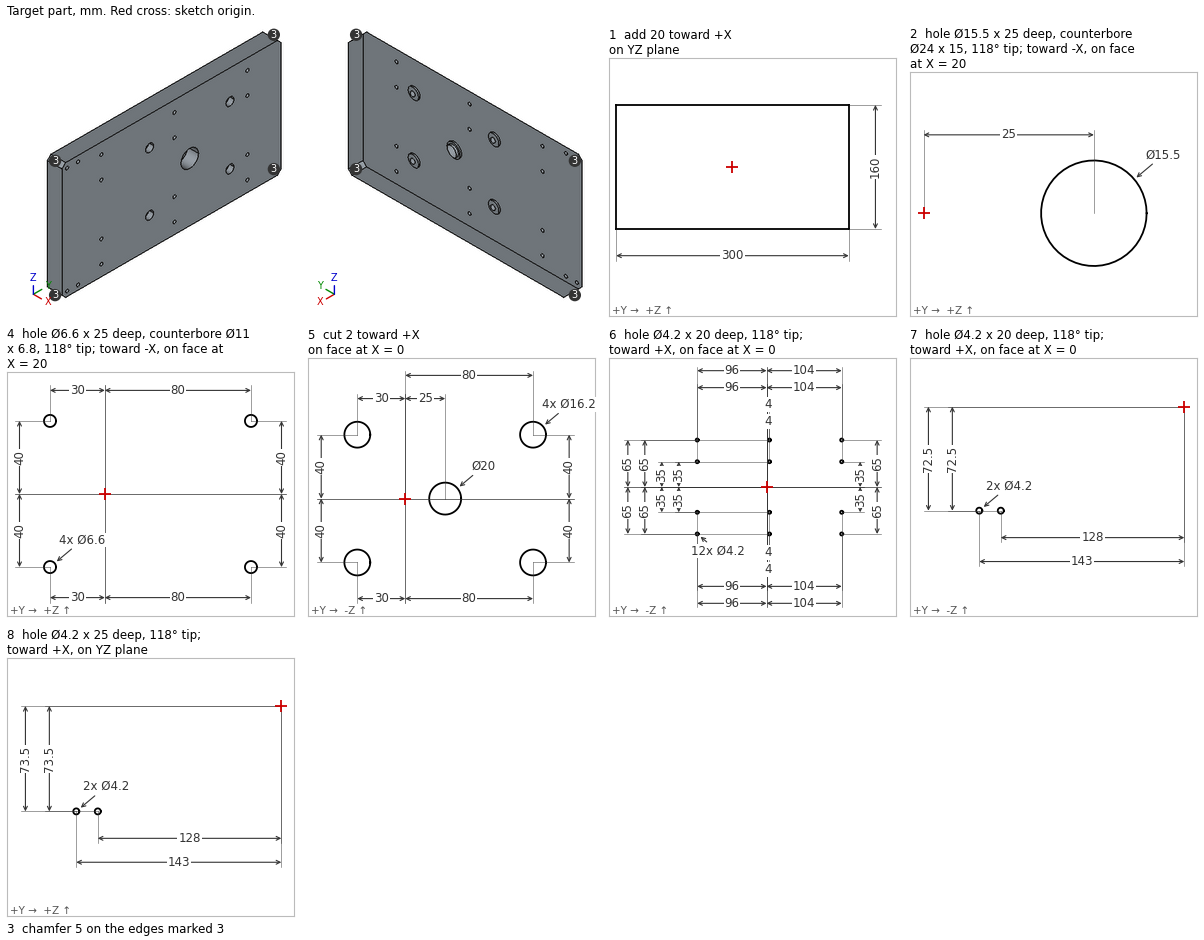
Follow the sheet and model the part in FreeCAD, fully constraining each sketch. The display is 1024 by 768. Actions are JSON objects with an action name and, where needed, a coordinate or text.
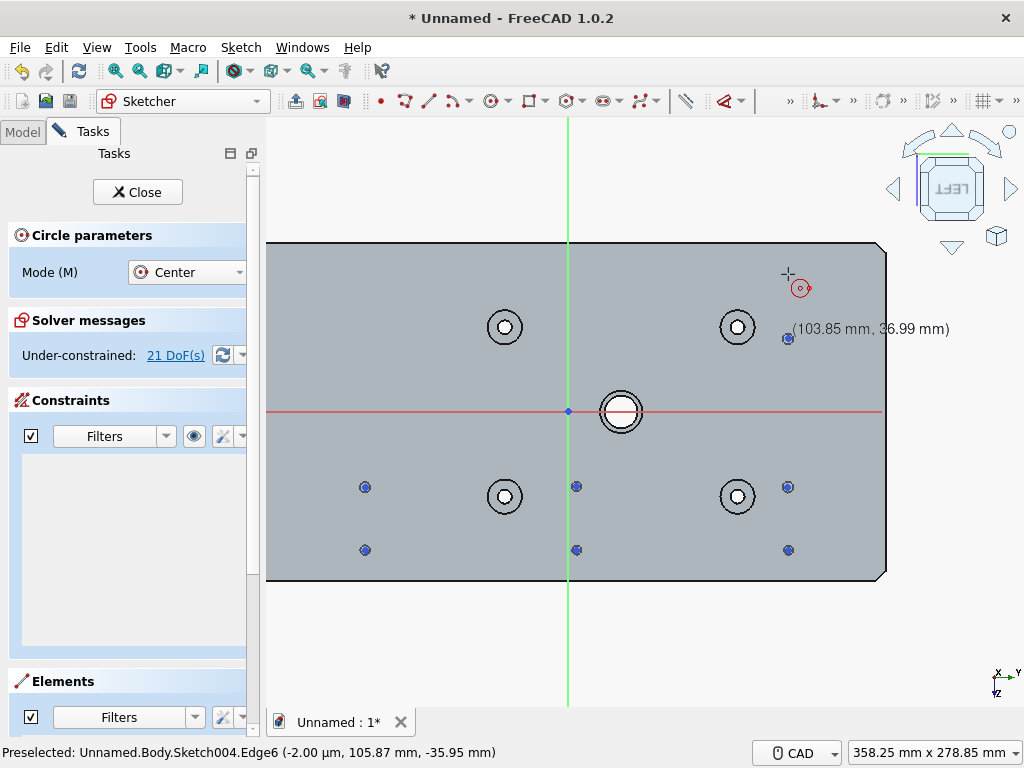
{"action": "left_click", "coordinate": [788, 274]}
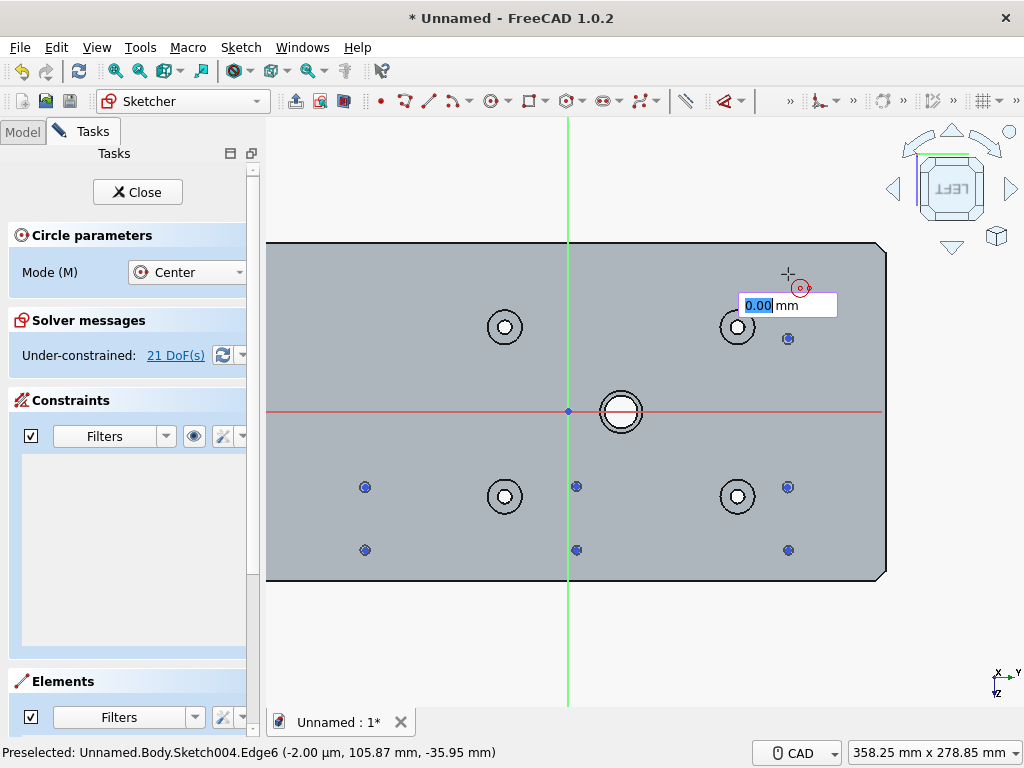
{"action": "scroll", "coordinate": [791, 271], "scroll_direction": "up", "scroll_amount": 7}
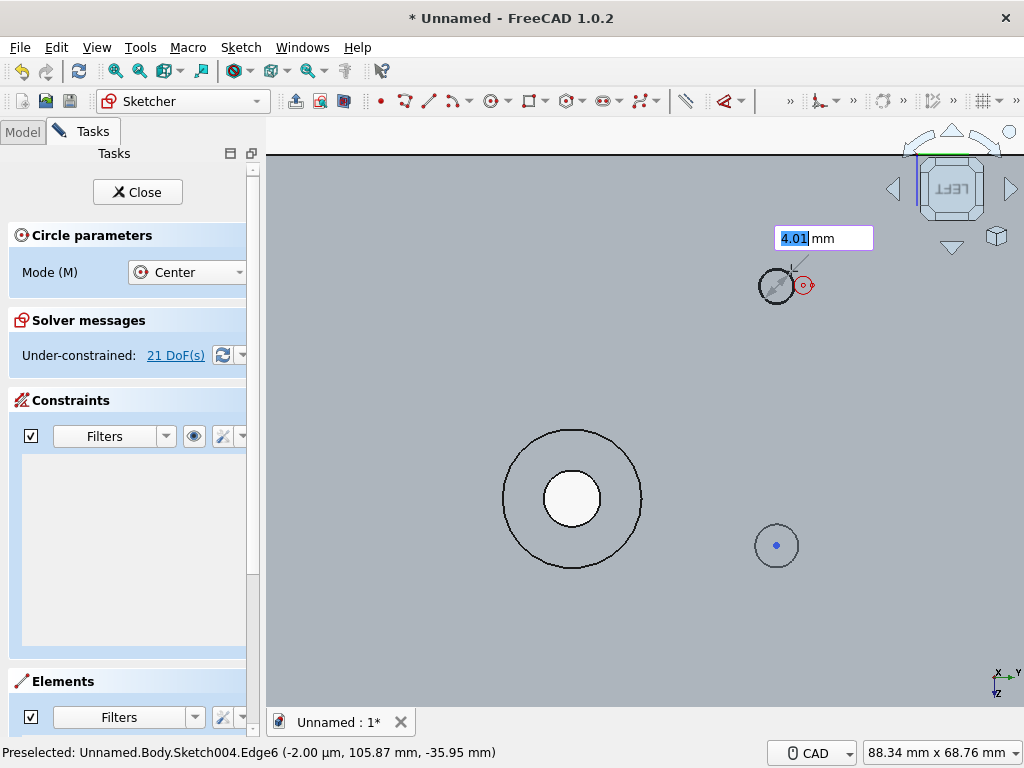
{"action": "left_click", "coordinate": [791, 271]}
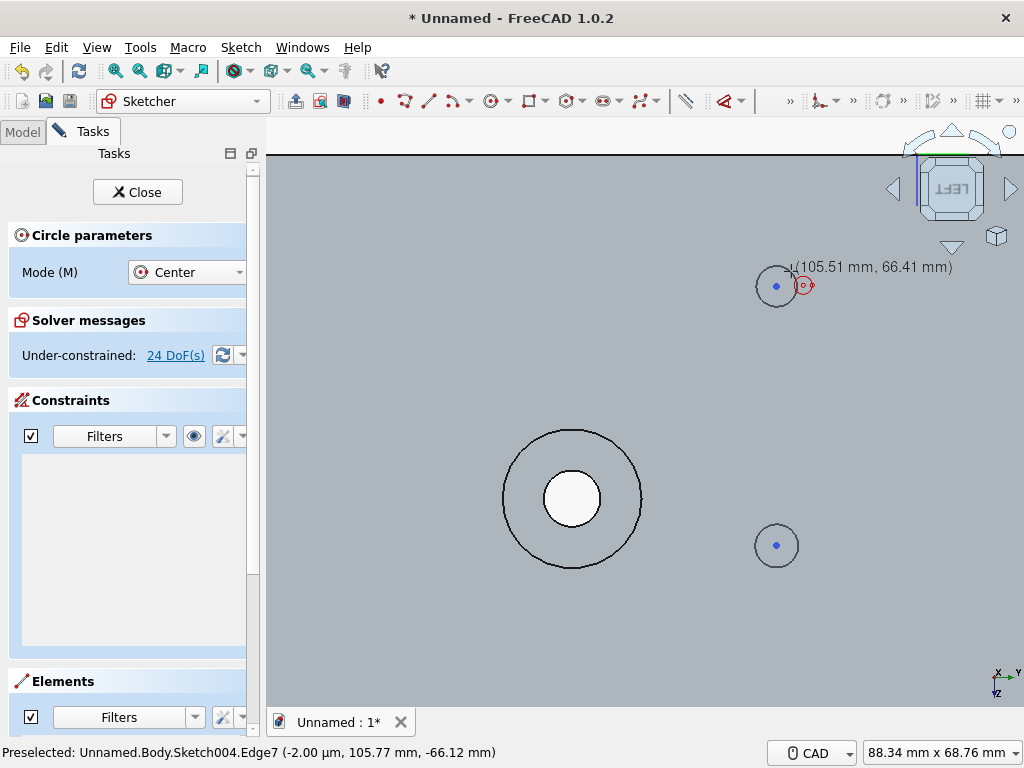
{"action": "scroll", "coordinate": [791, 271], "scroll_direction": "down", "scroll_amount": 7}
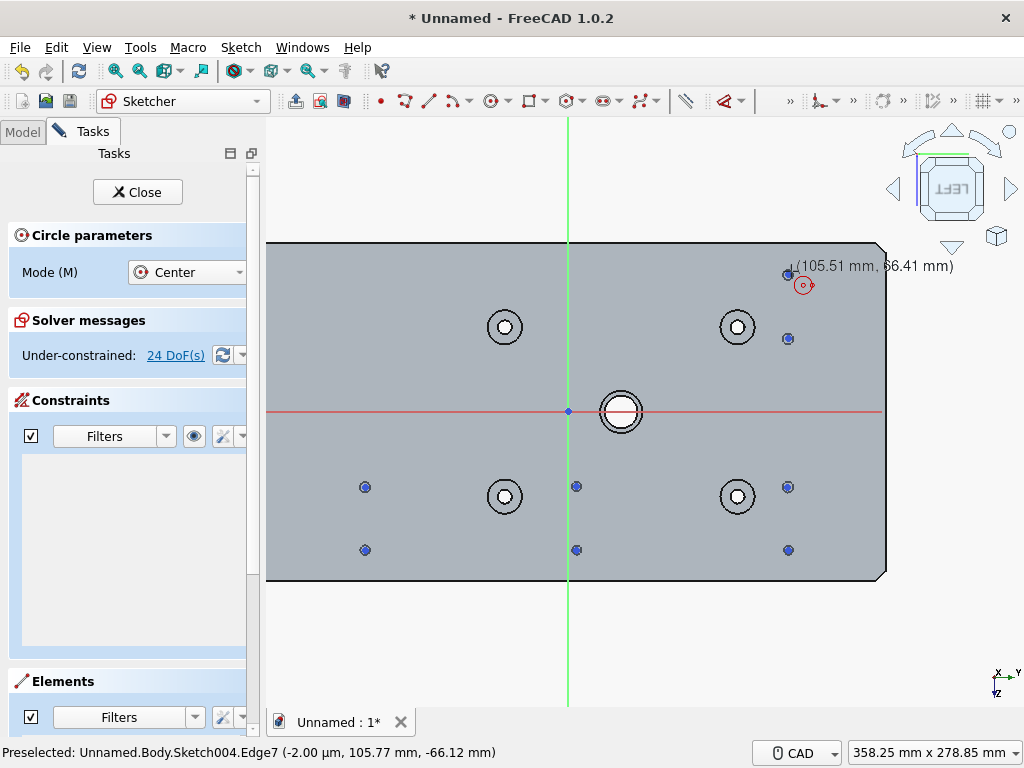
{"action": "scroll", "coordinate": [577, 338], "scroll_direction": "up", "scroll_amount": 9}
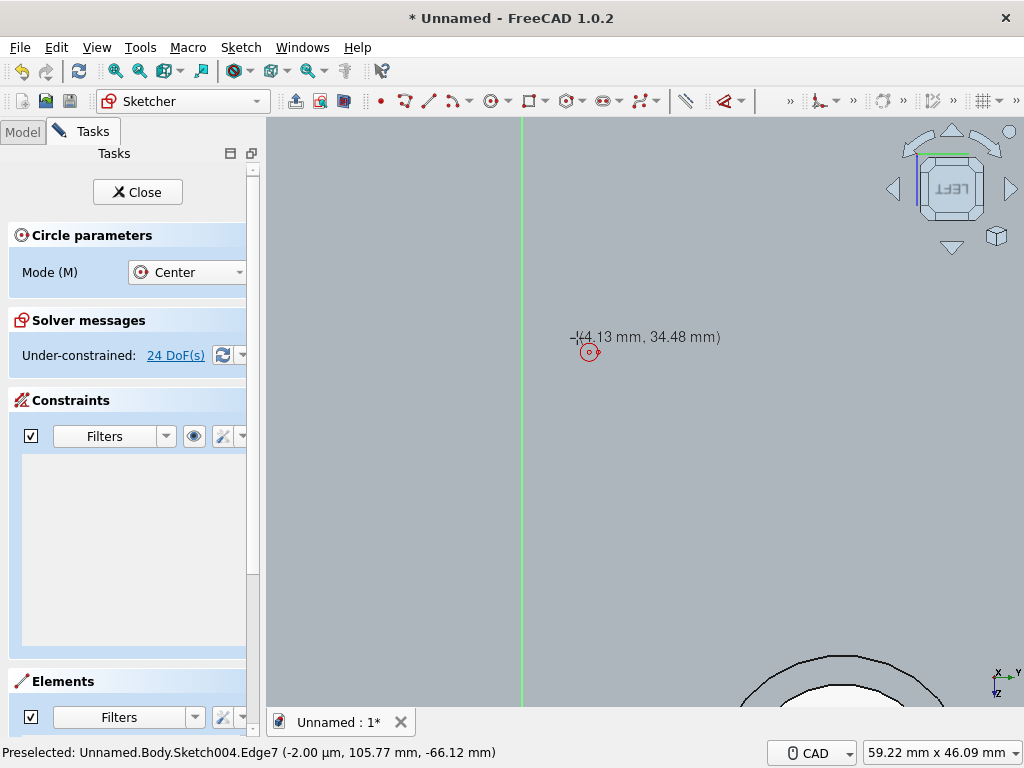
{"action": "scroll", "coordinate": [577, 338], "scroll_direction": "down", "scroll_amount": 9}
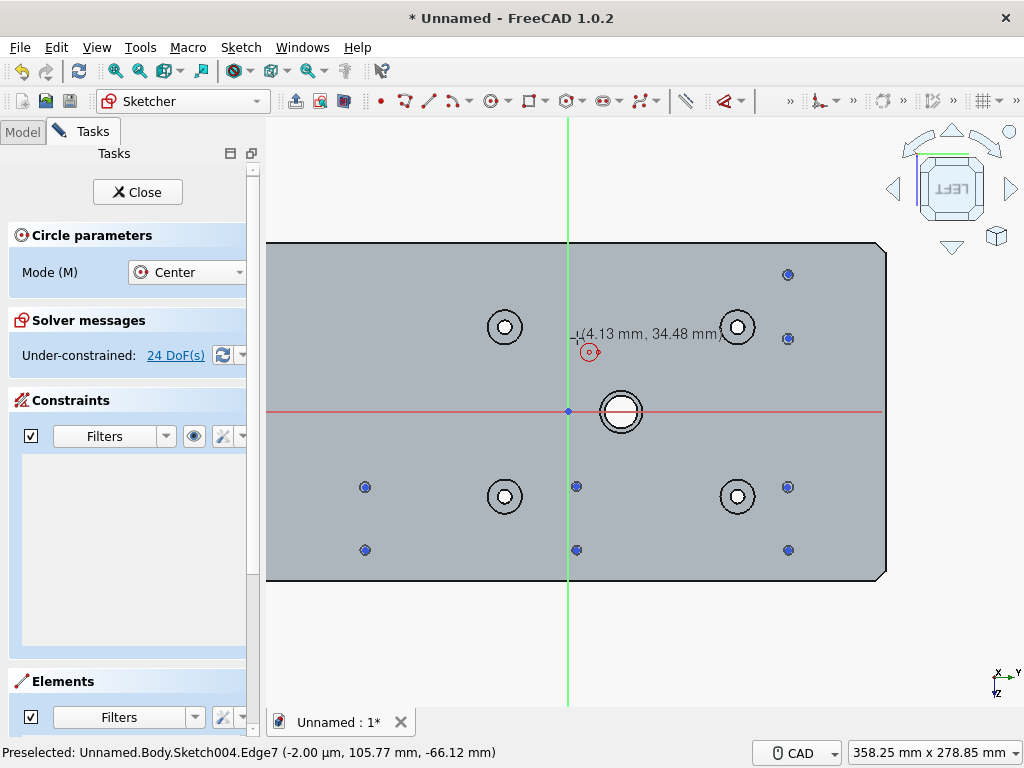
{"action": "scroll", "coordinate": [577, 338], "scroll_direction": "up", "scroll_amount": 4}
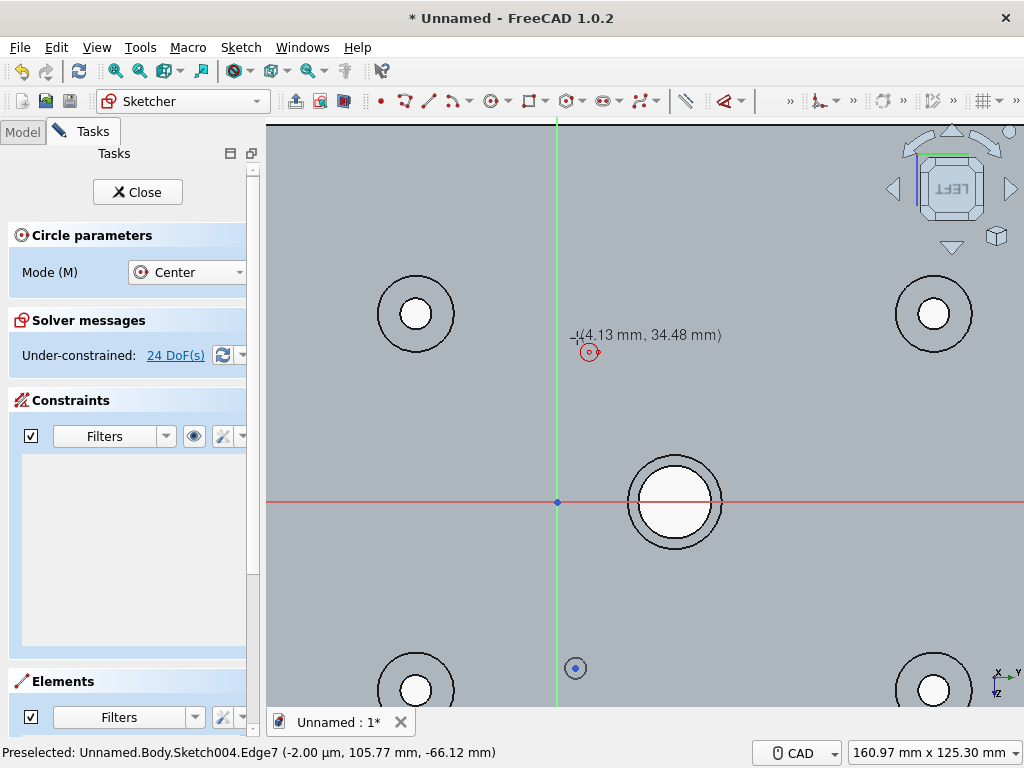
{"action": "left_click", "coordinate": [576, 337]}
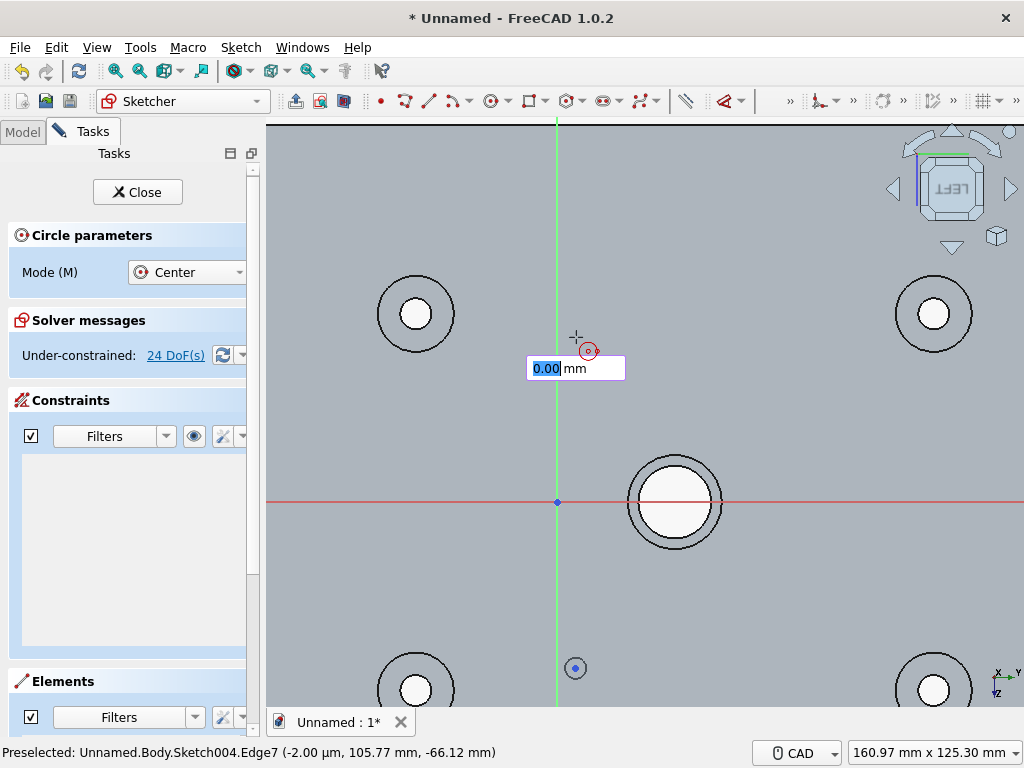
{"action": "scroll", "coordinate": [583, 330], "scroll_direction": "up", "scroll_amount": 3}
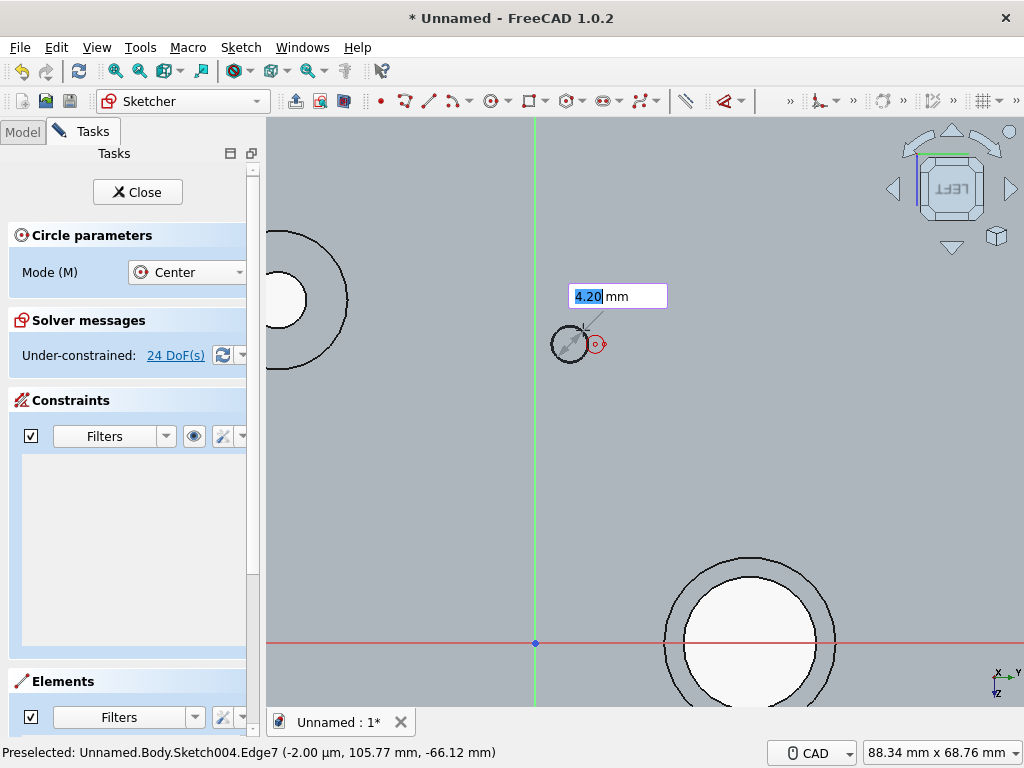
{"action": "left_click", "coordinate": [582, 330]}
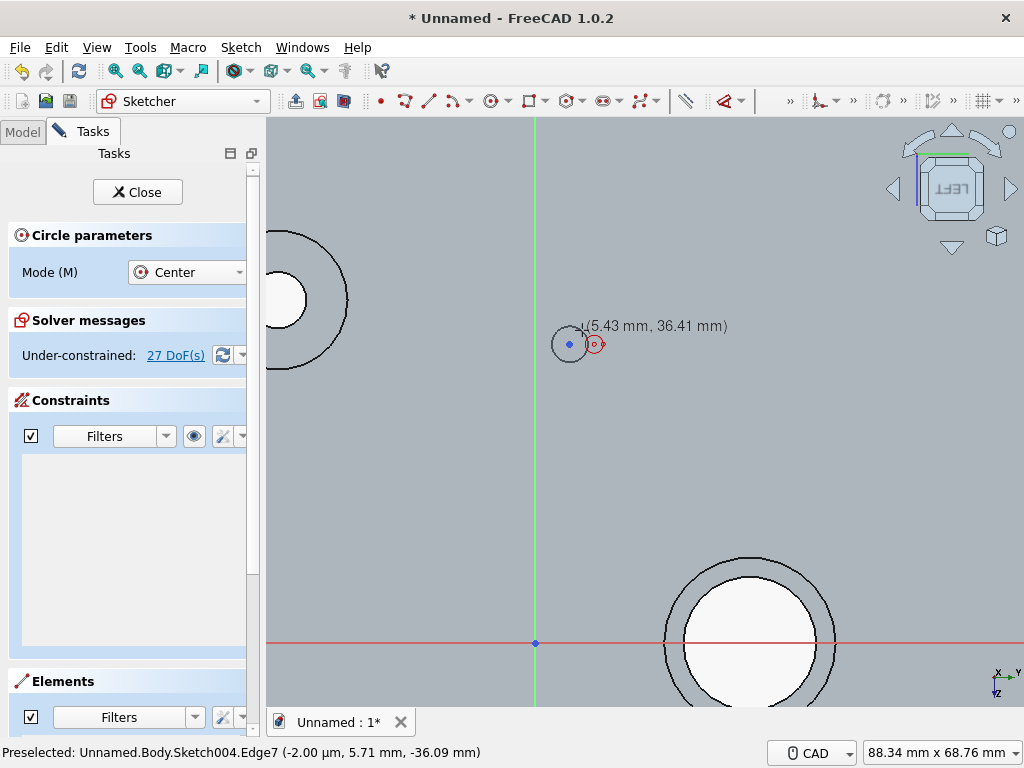
{"action": "scroll", "coordinate": [579, 336], "scroll_direction": "down", "scroll_amount": 7}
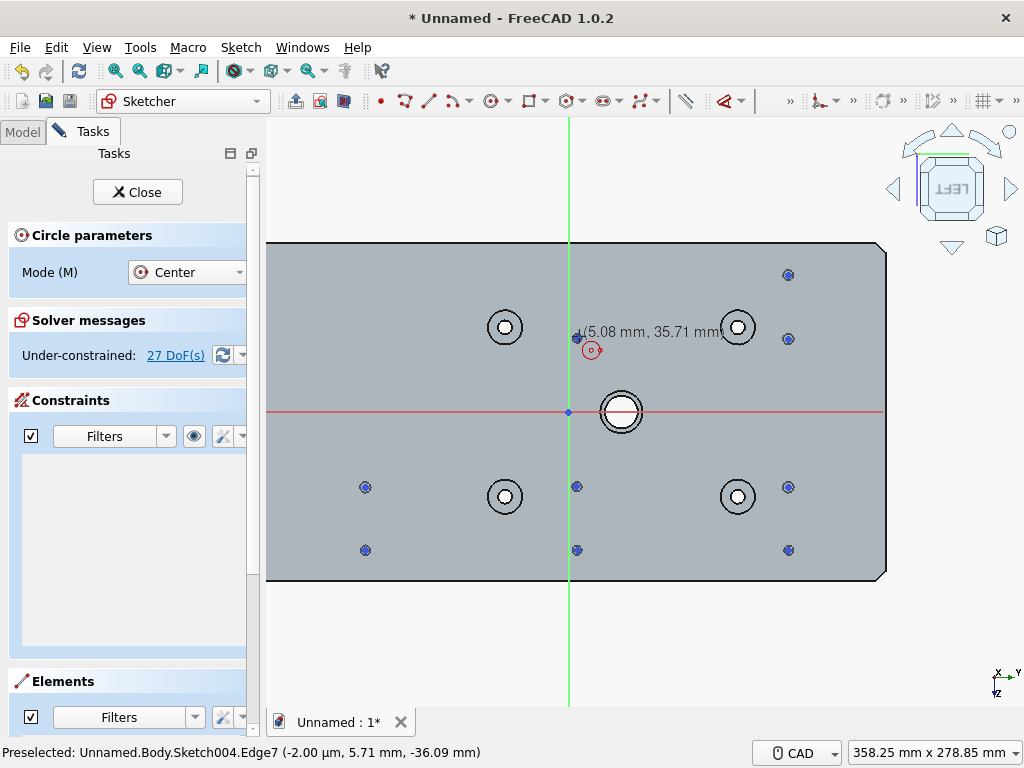
{"action": "scroll", "coordinate": [577, 275], "scroll_direction": "up", "scroll_amount": 9}